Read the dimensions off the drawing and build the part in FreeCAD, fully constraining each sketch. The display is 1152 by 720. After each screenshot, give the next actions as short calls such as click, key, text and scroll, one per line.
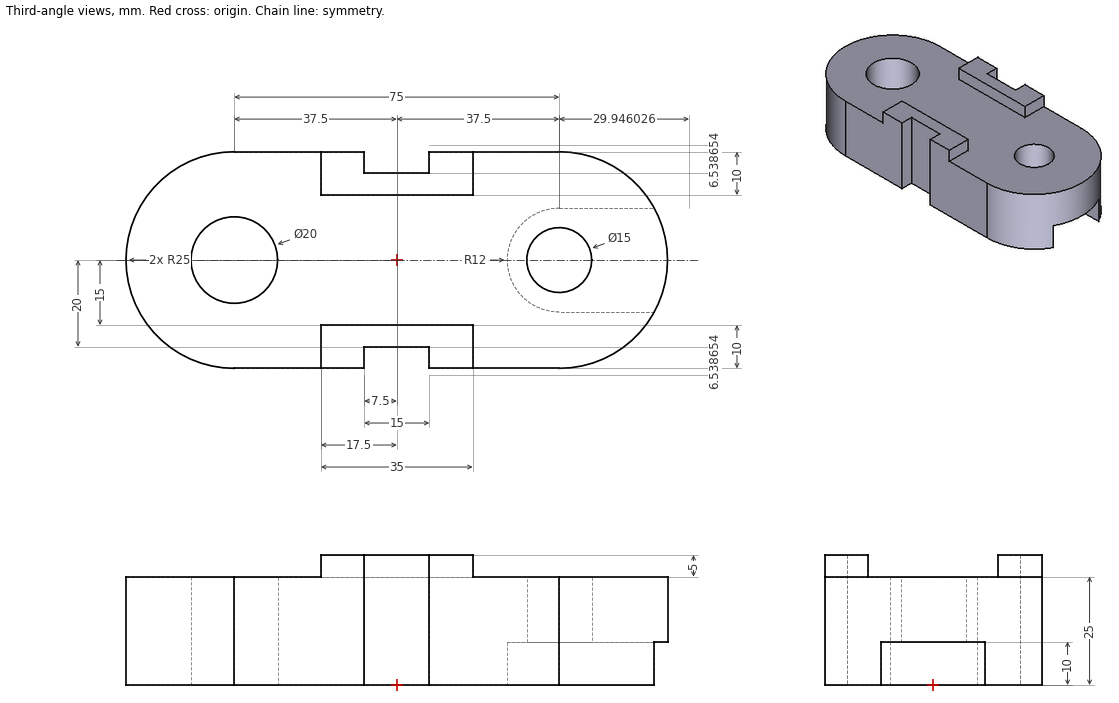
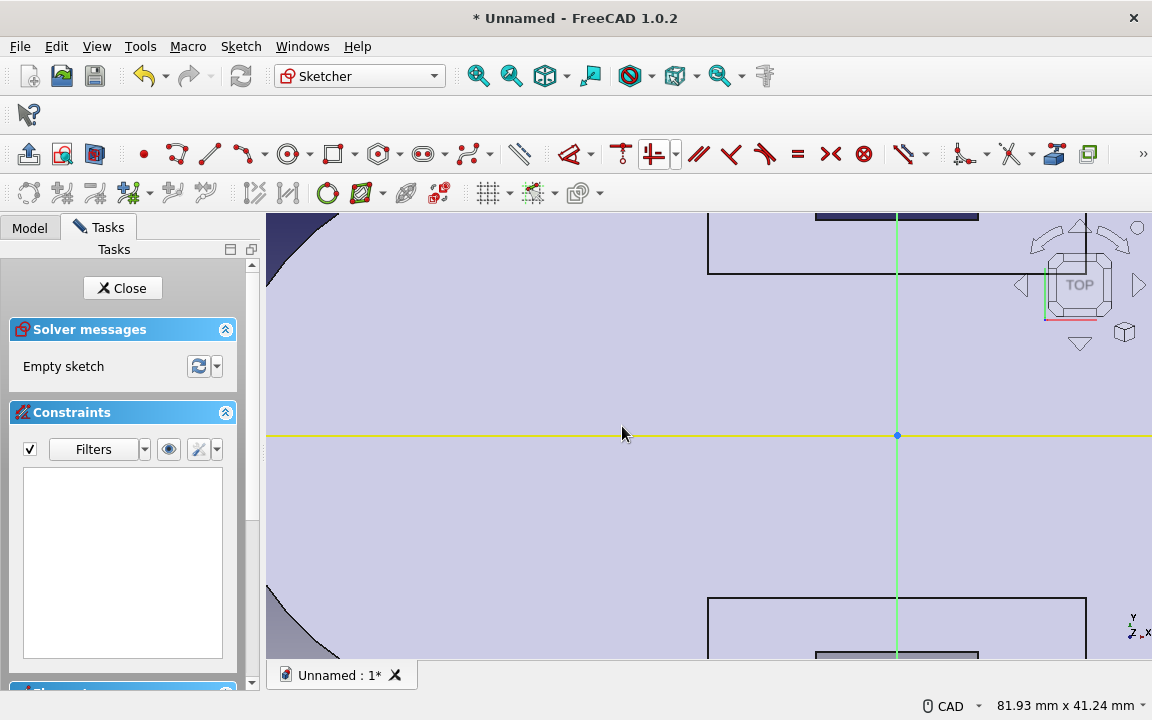
click(288, 154)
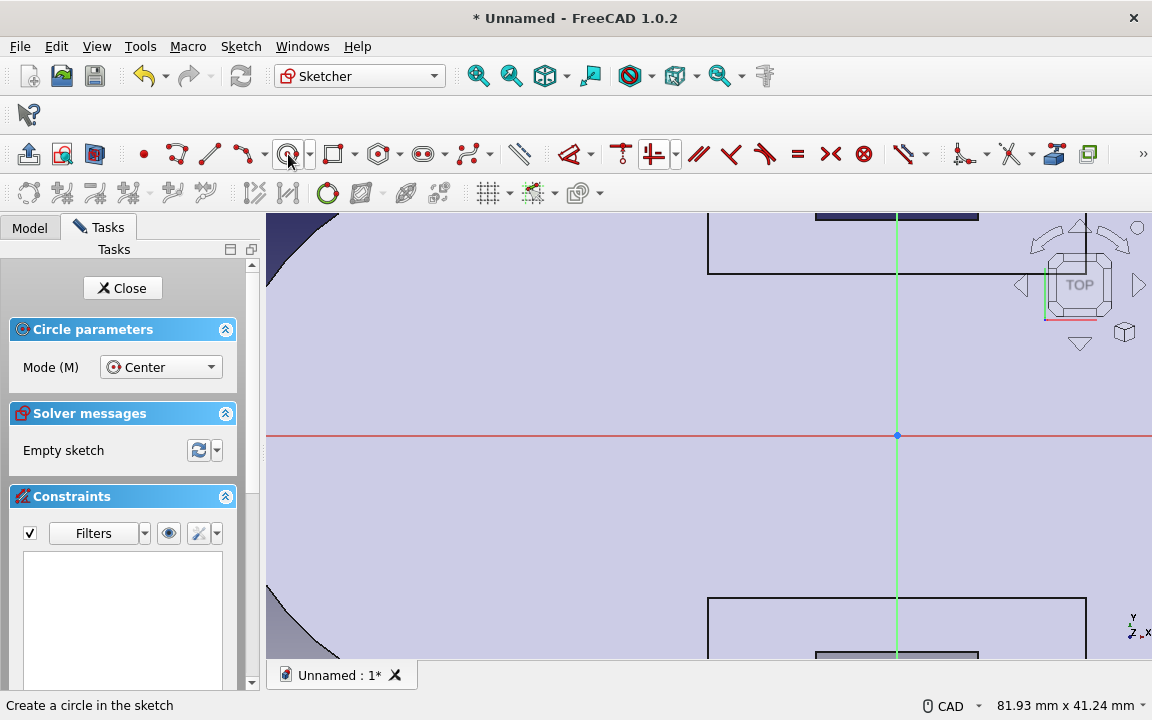
click(492, 436)
move(568, 359)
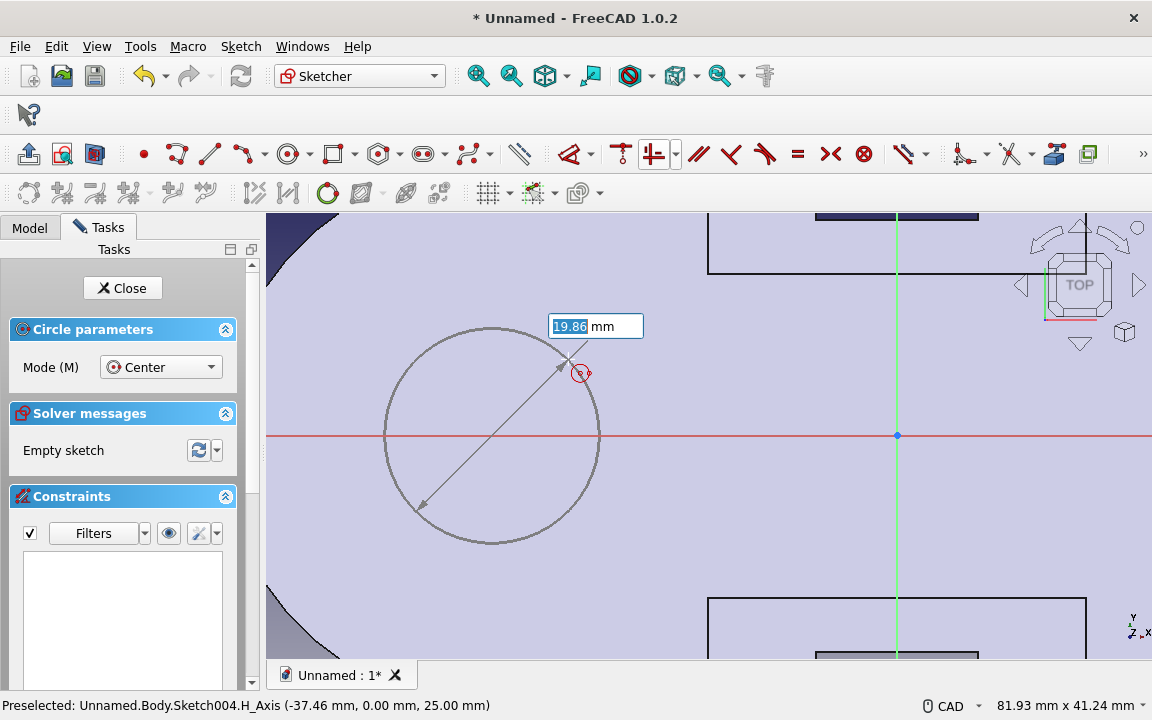
text(20)
key(Return)
key(Escape)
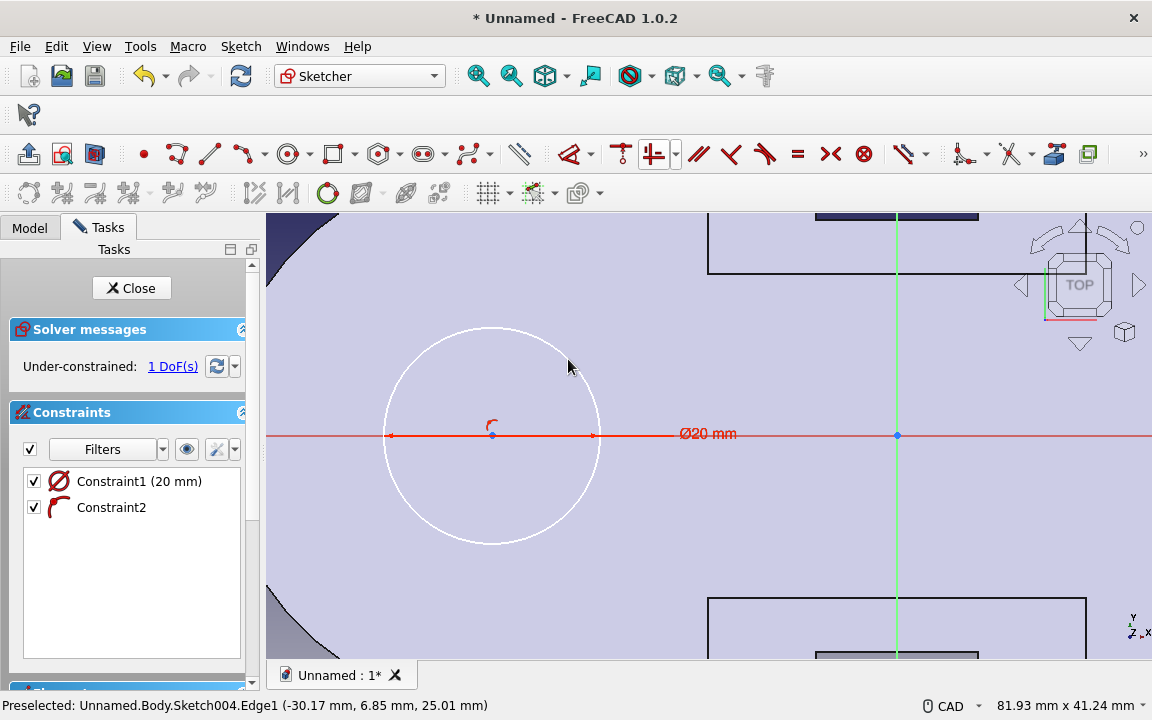
click(568, 154)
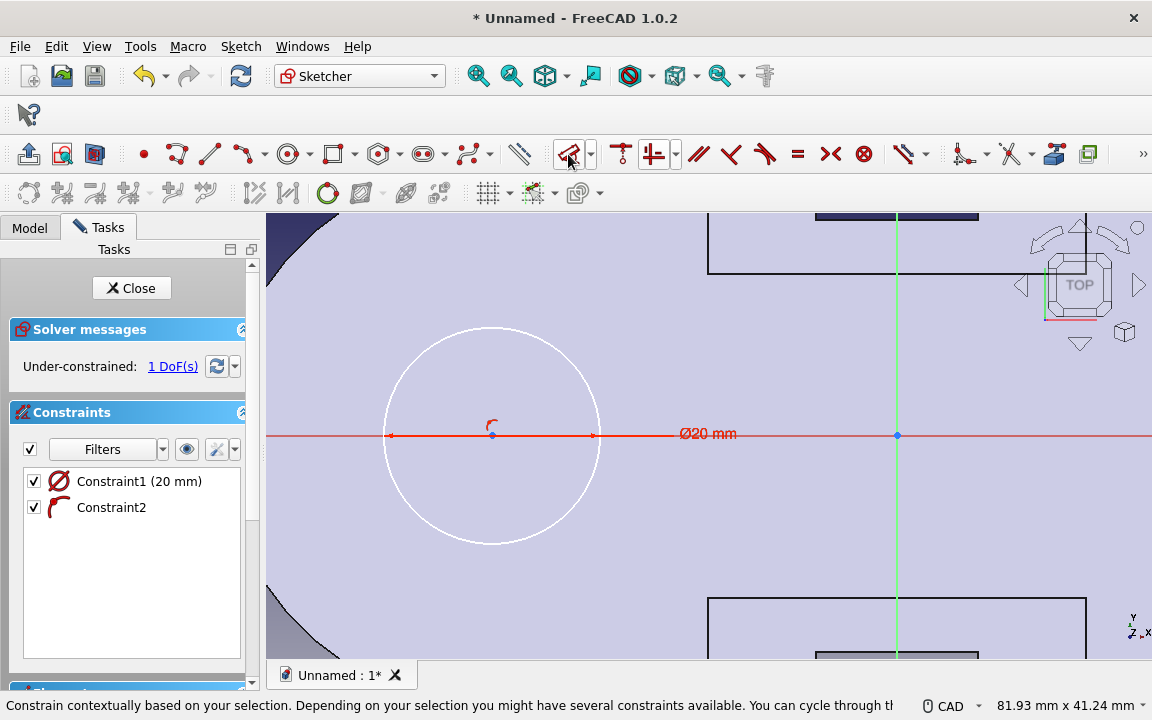
click(492, 436)
click(695, 470)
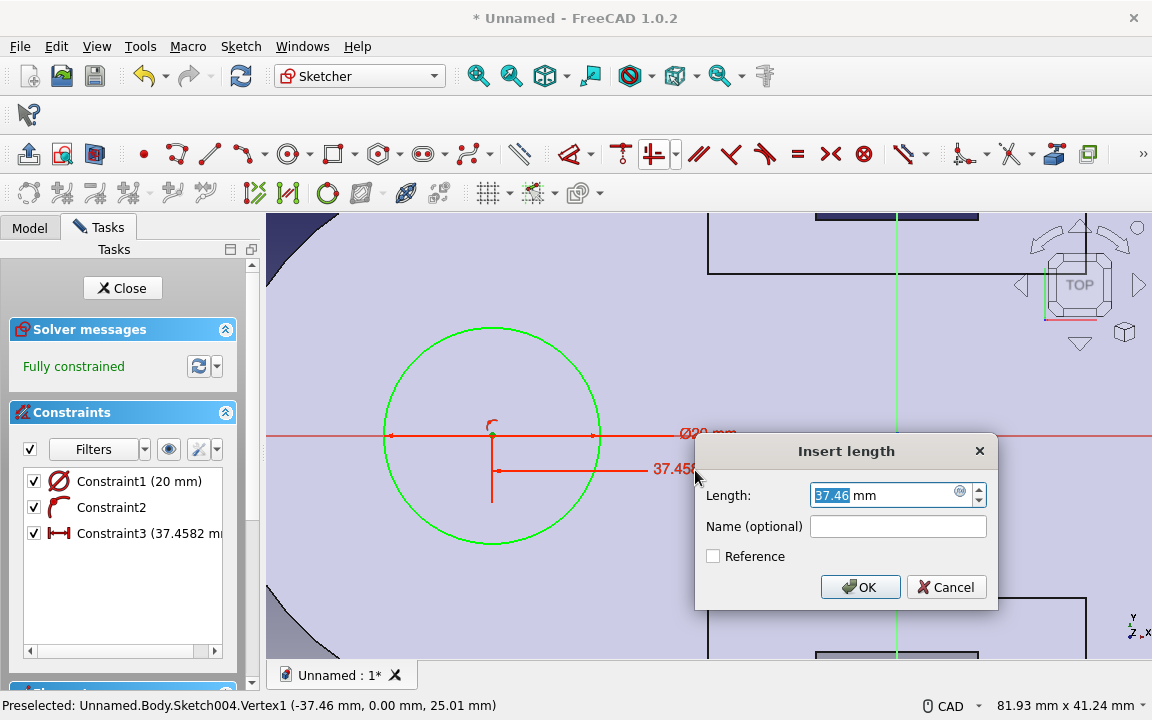
text(37.5)
key(Return)
key(Escape)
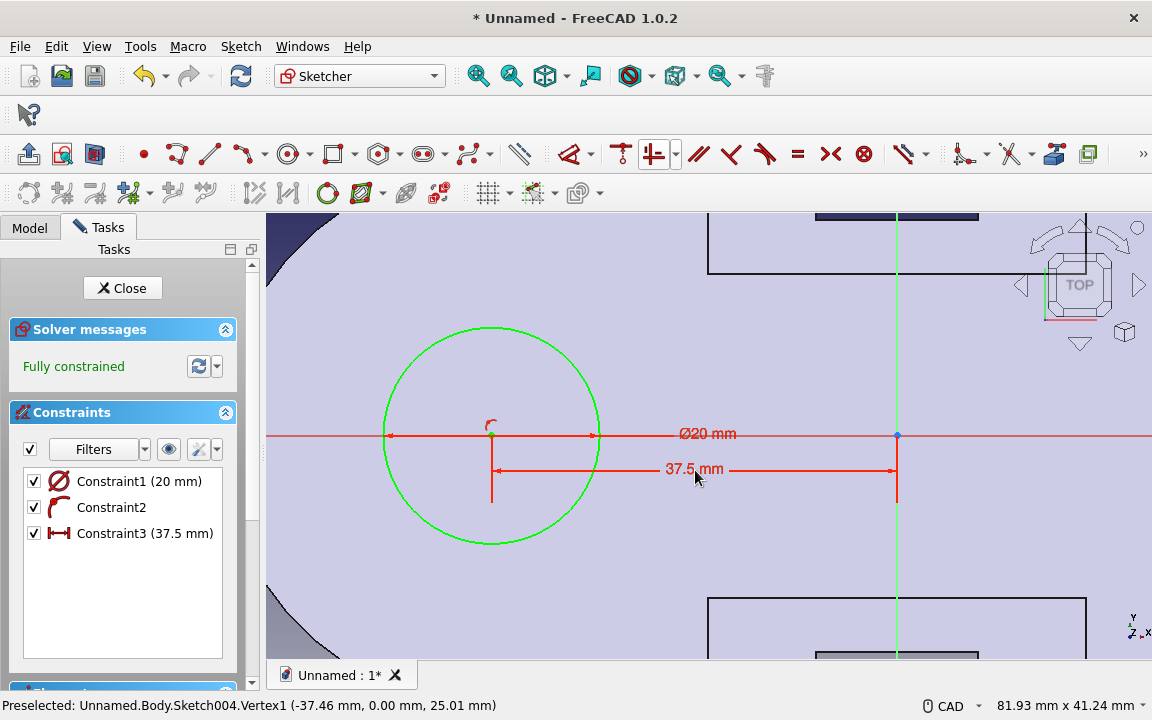
click(123, 288)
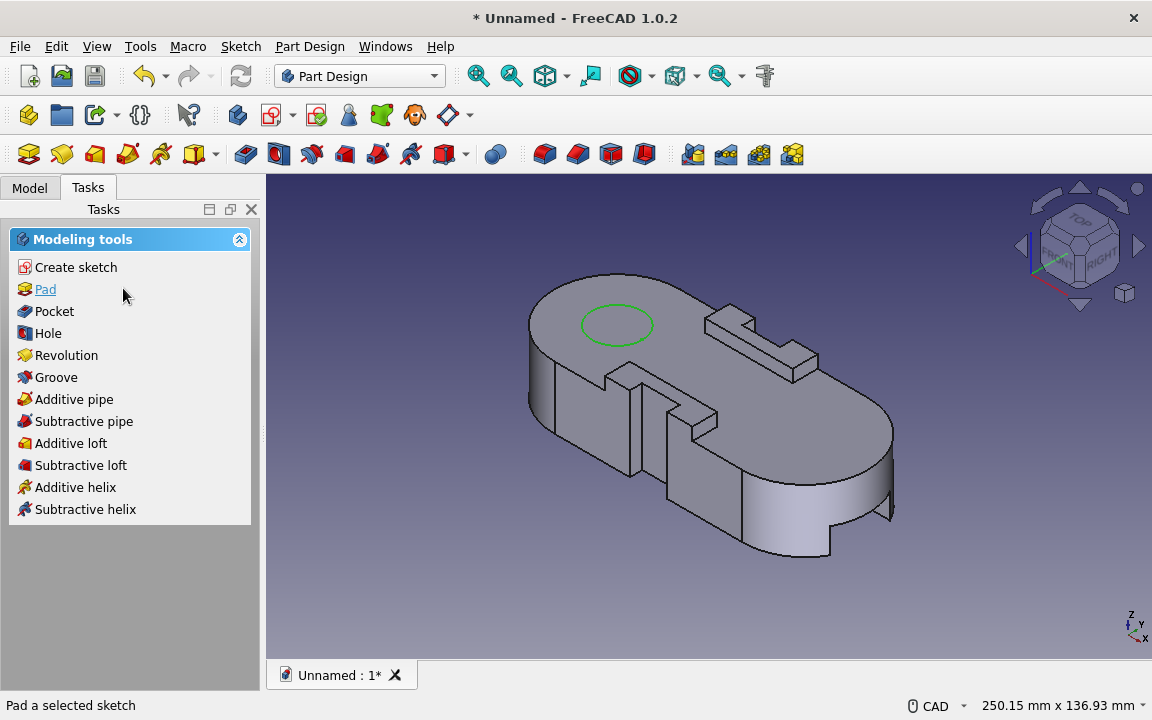
click(246, 154)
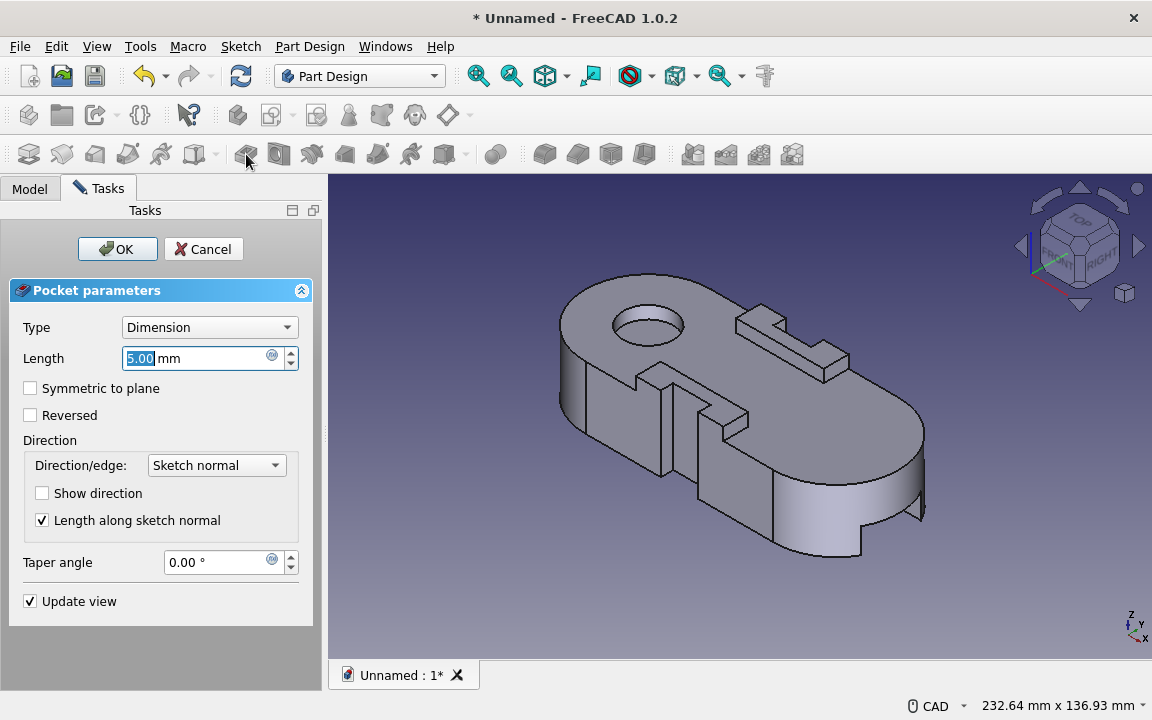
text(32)
key(Tab)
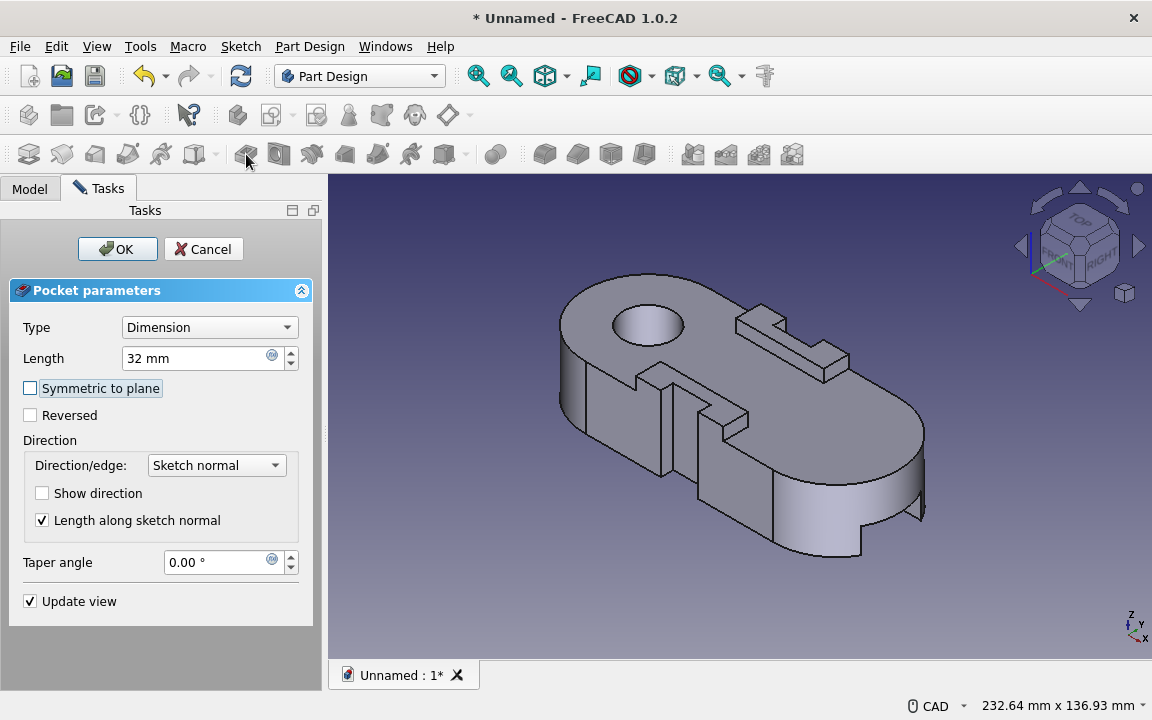
click(118, 249)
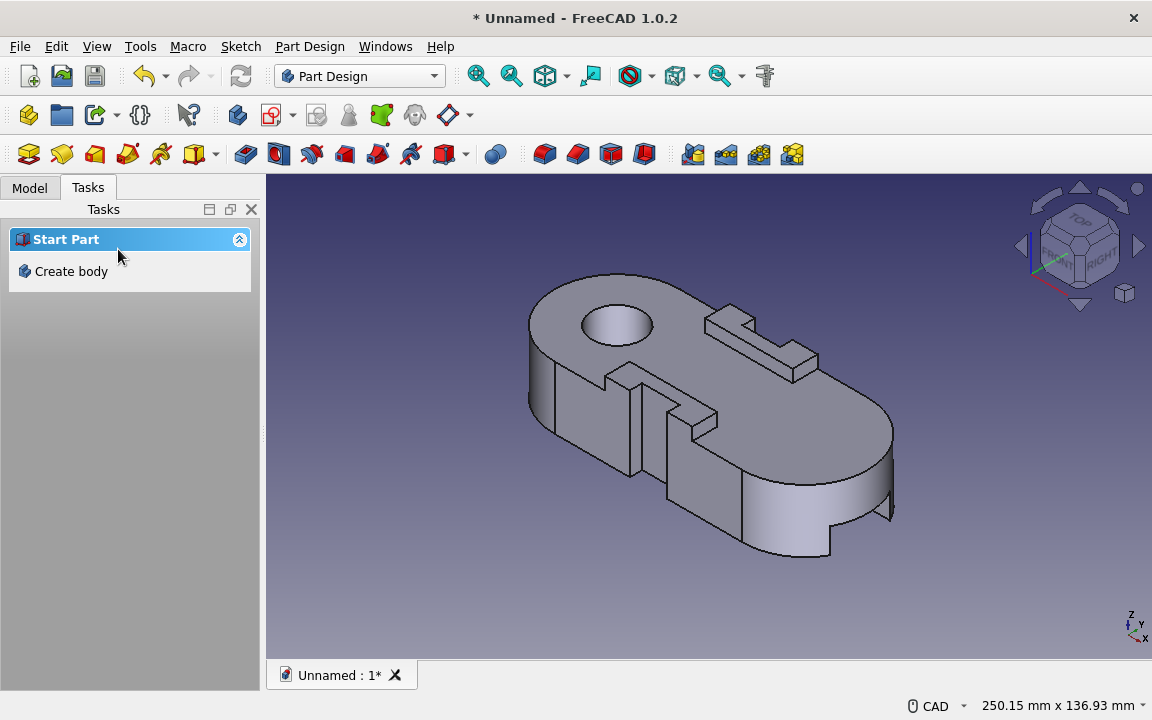
click(801, 430)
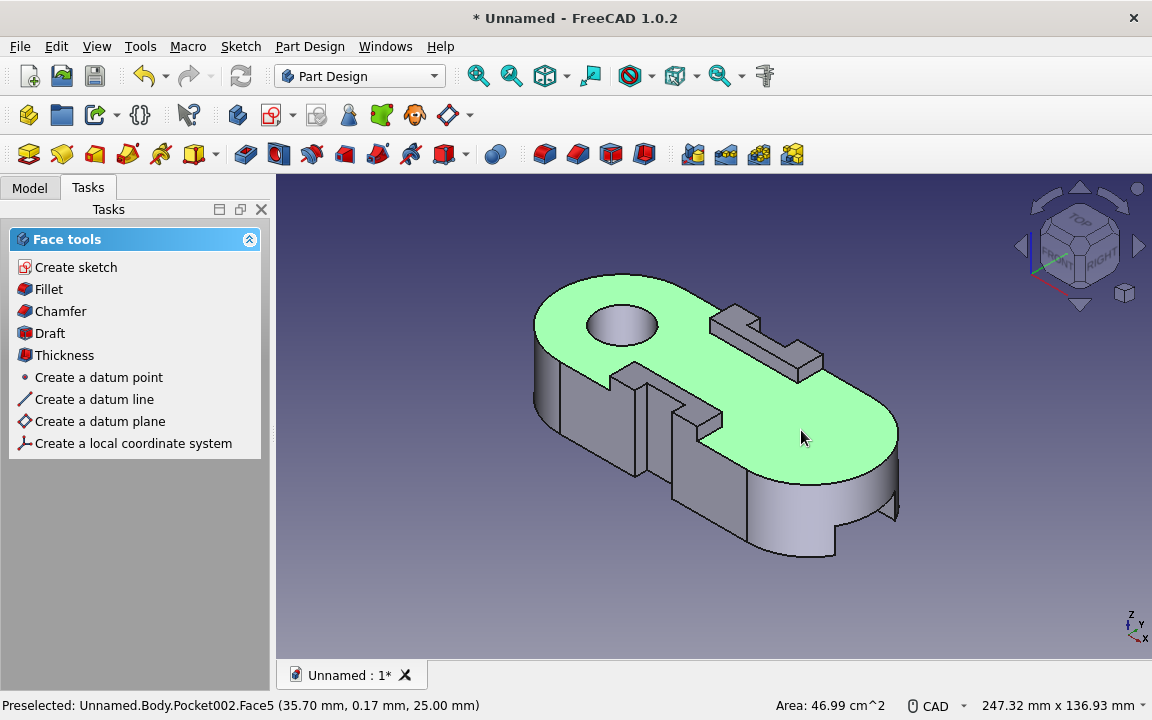
click(270, 116)